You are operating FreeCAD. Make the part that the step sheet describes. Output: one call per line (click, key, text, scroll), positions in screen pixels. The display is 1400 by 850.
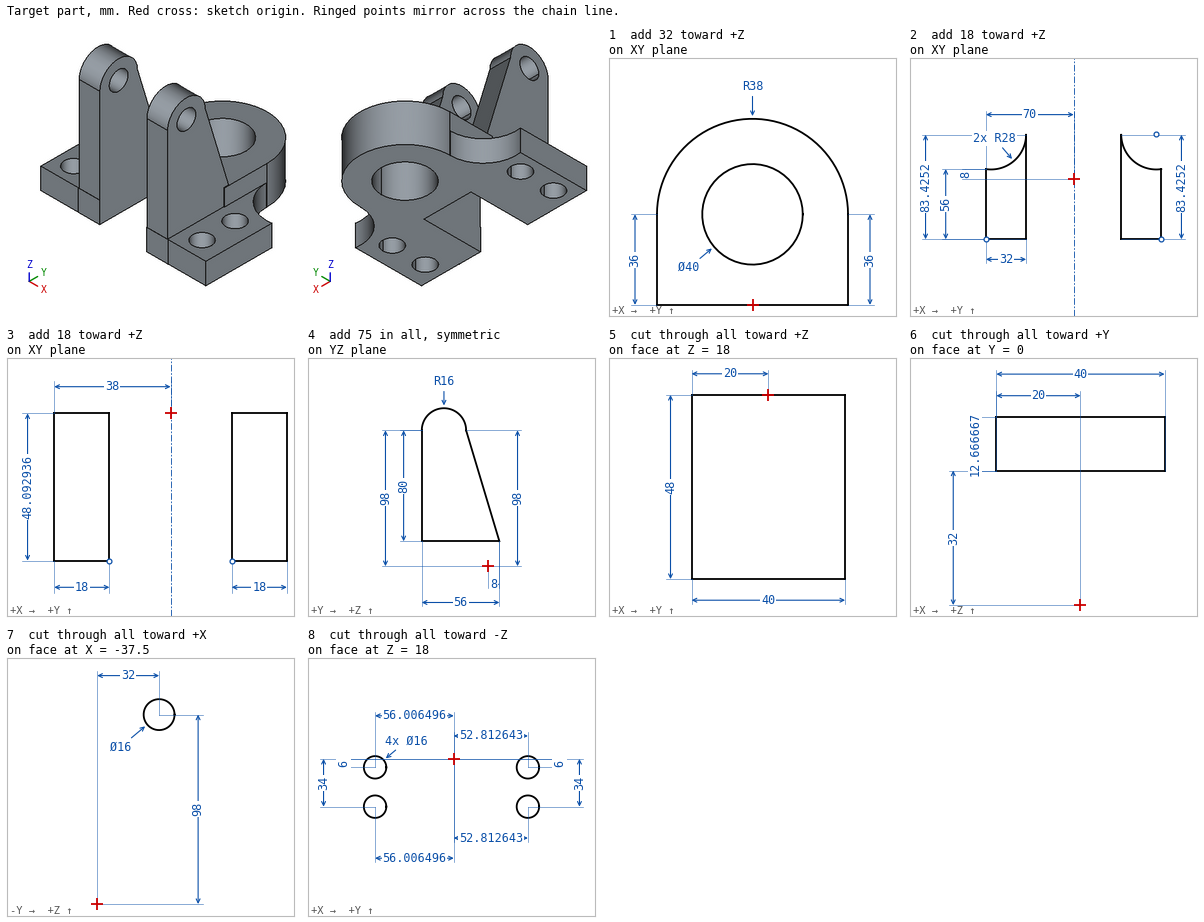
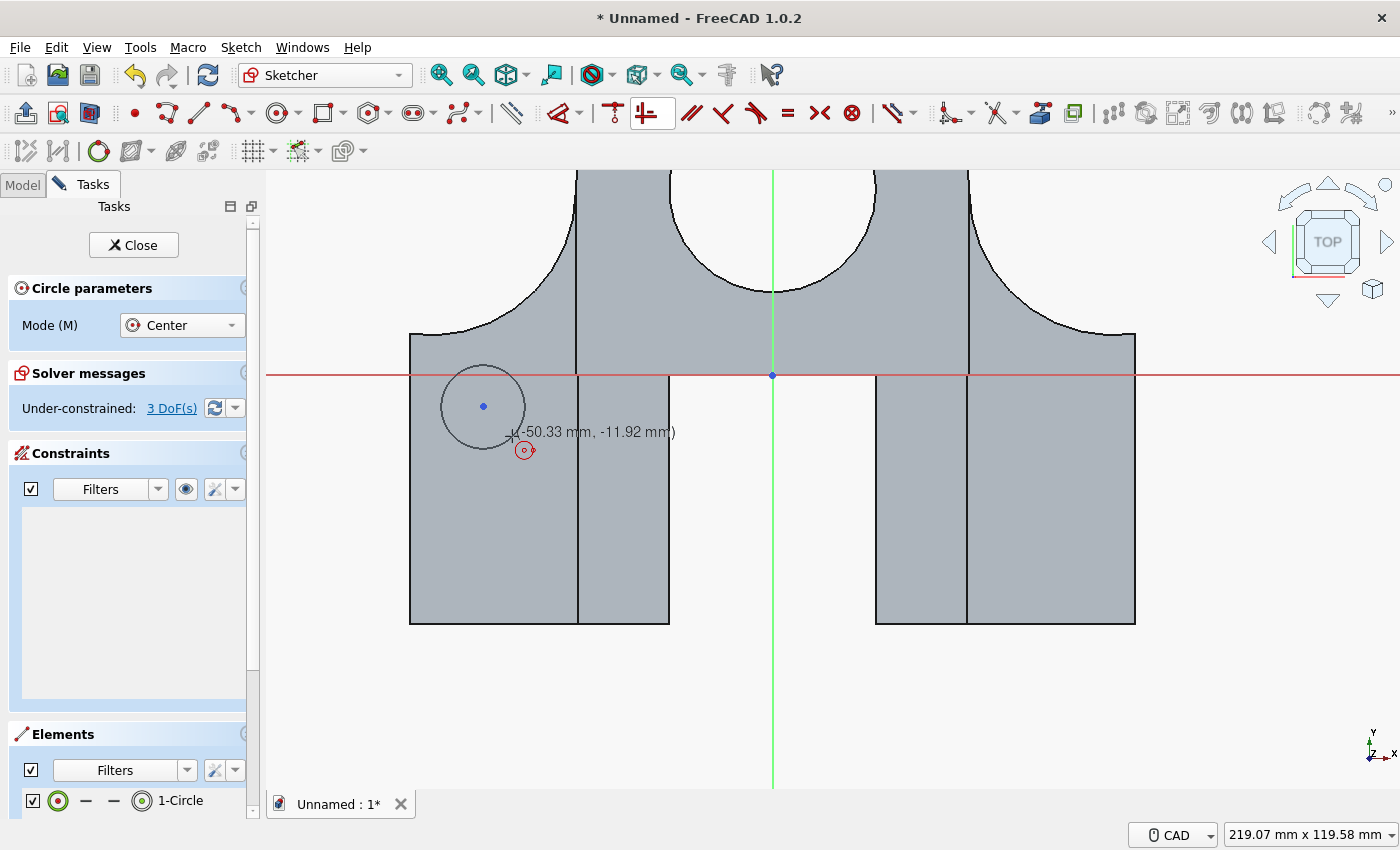
click(483, 551)
click(512, 522)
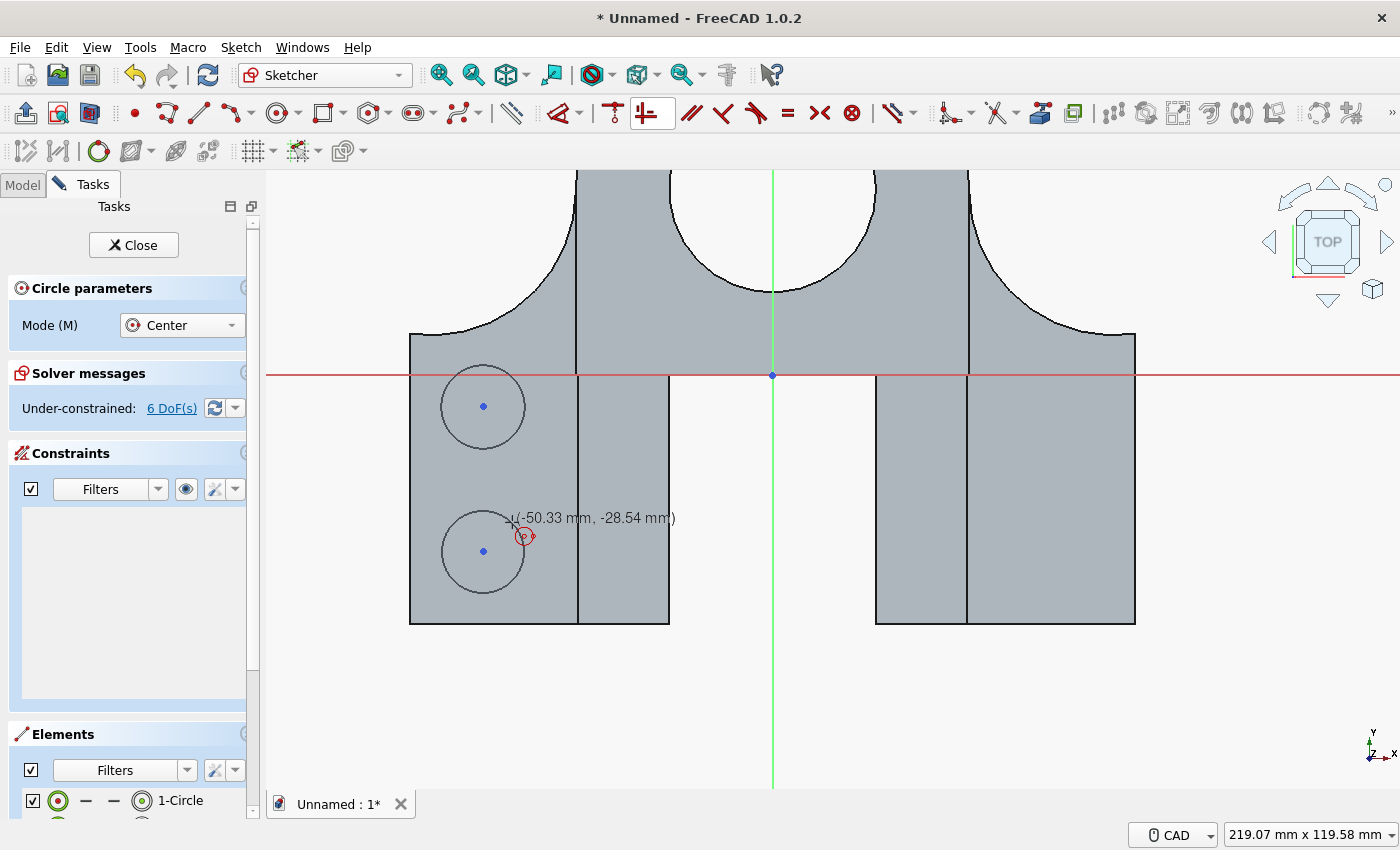
click(1046, 406)
click(1075, 436)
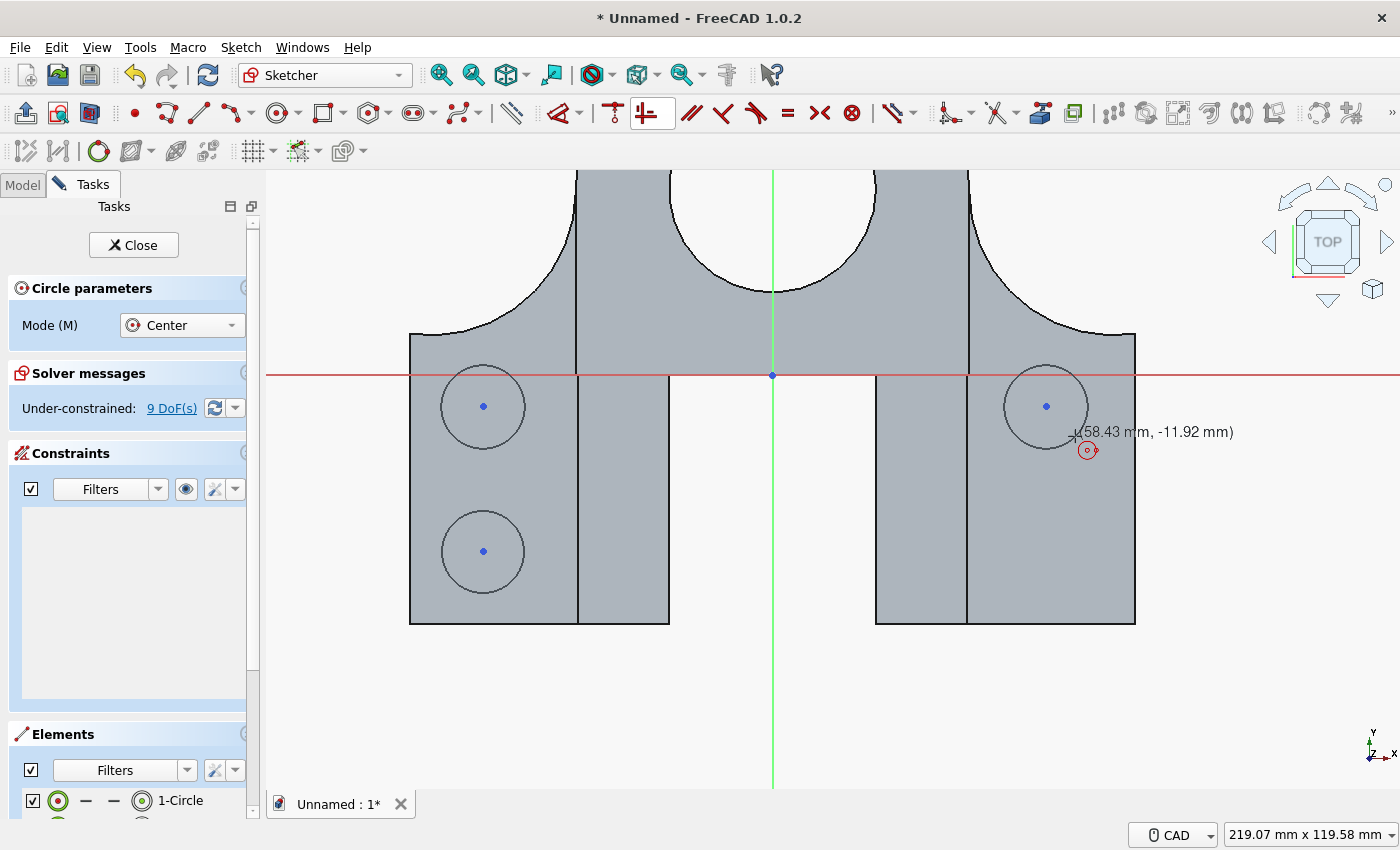
click(1046, 551)
click(1075, 522)
key(Escape)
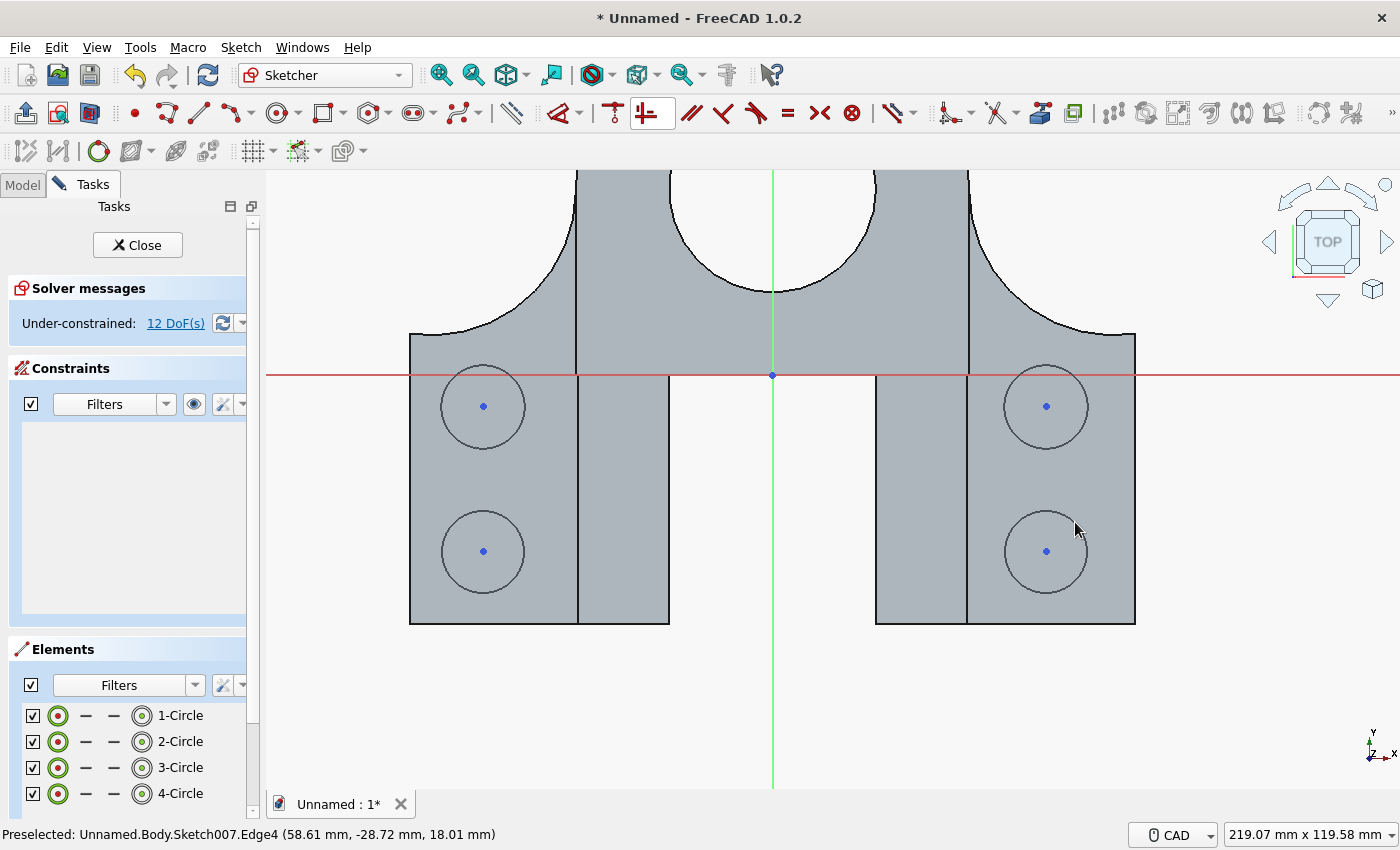
click(512, 377)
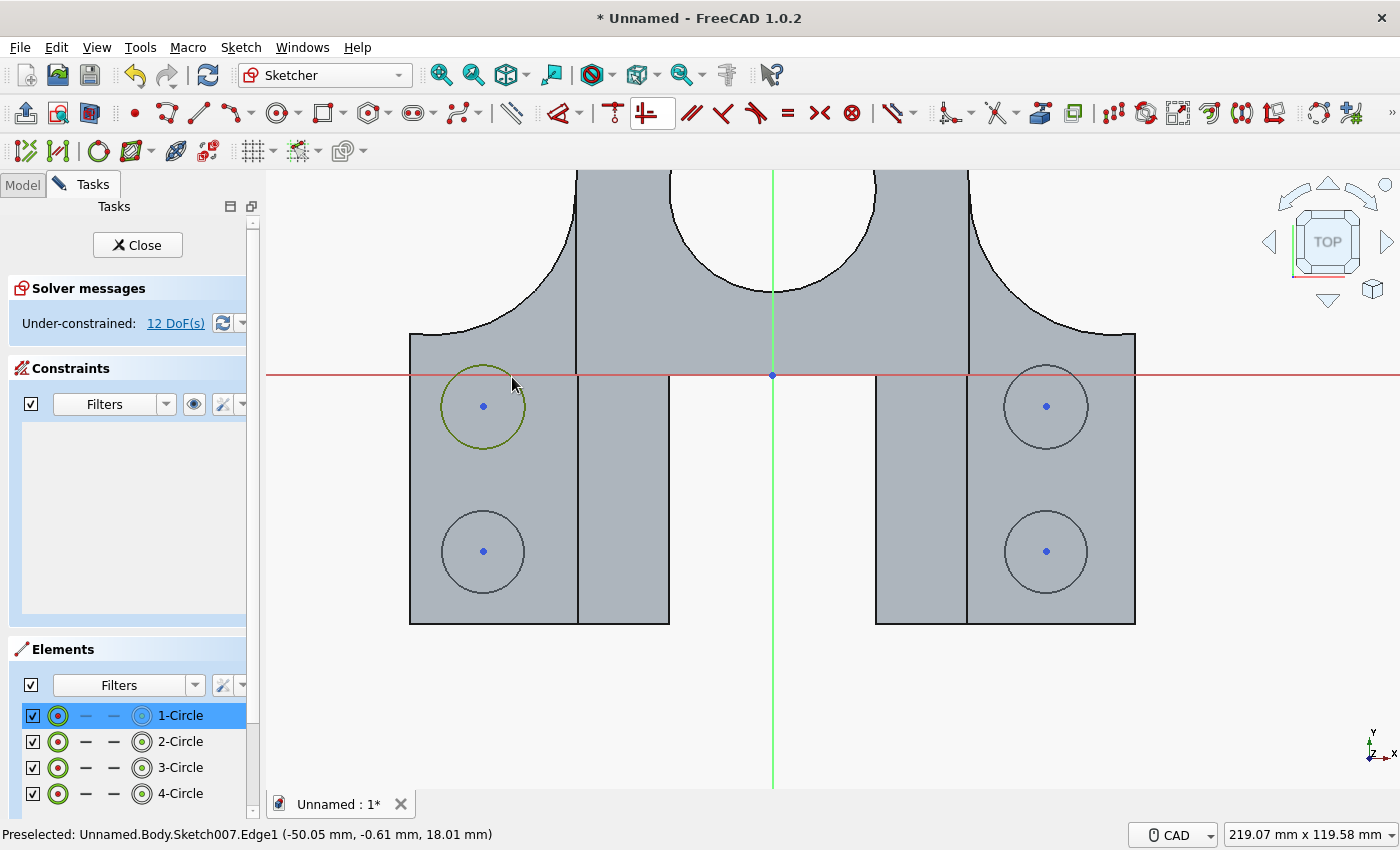
click(512, 523)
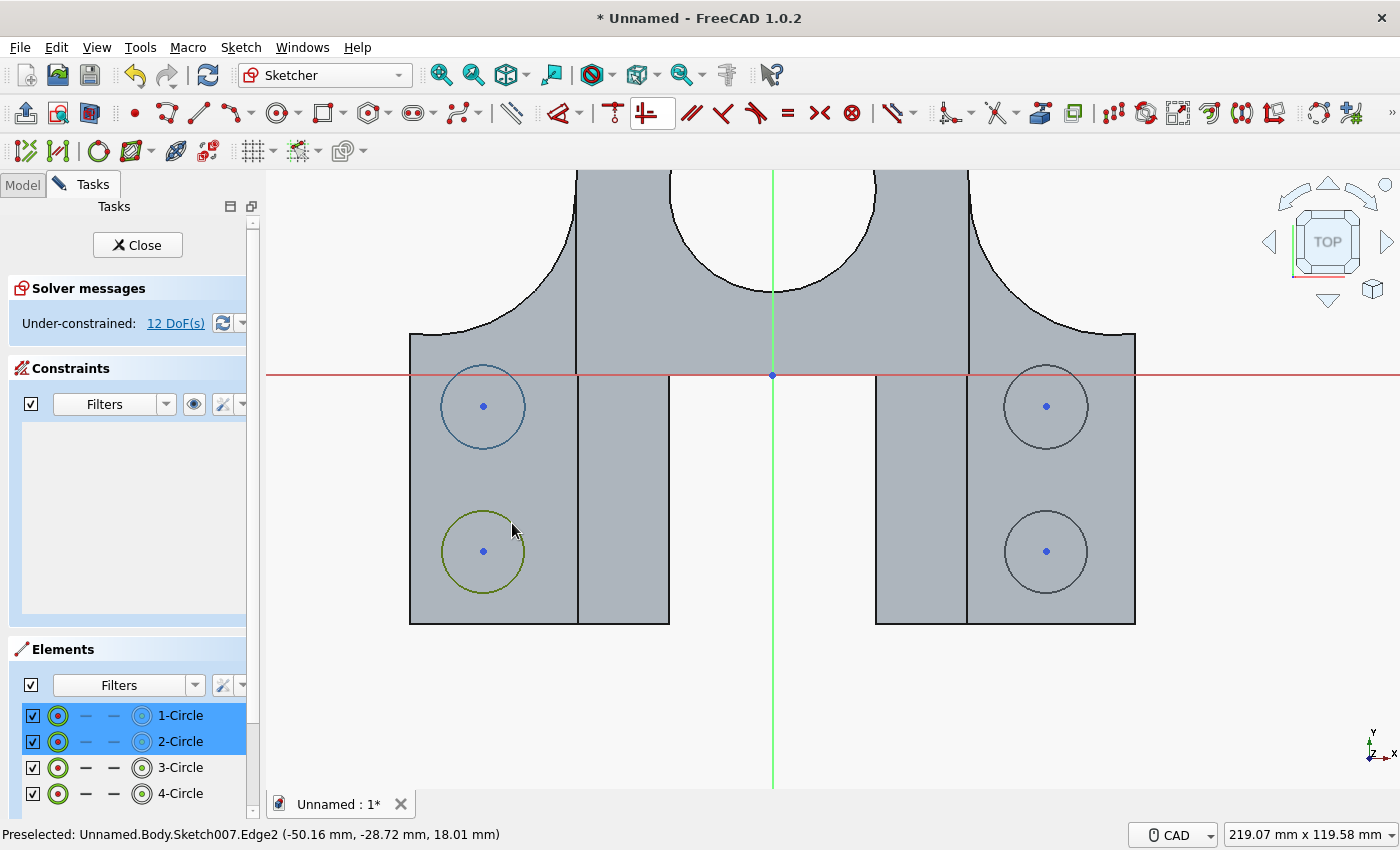
click(1075, 377)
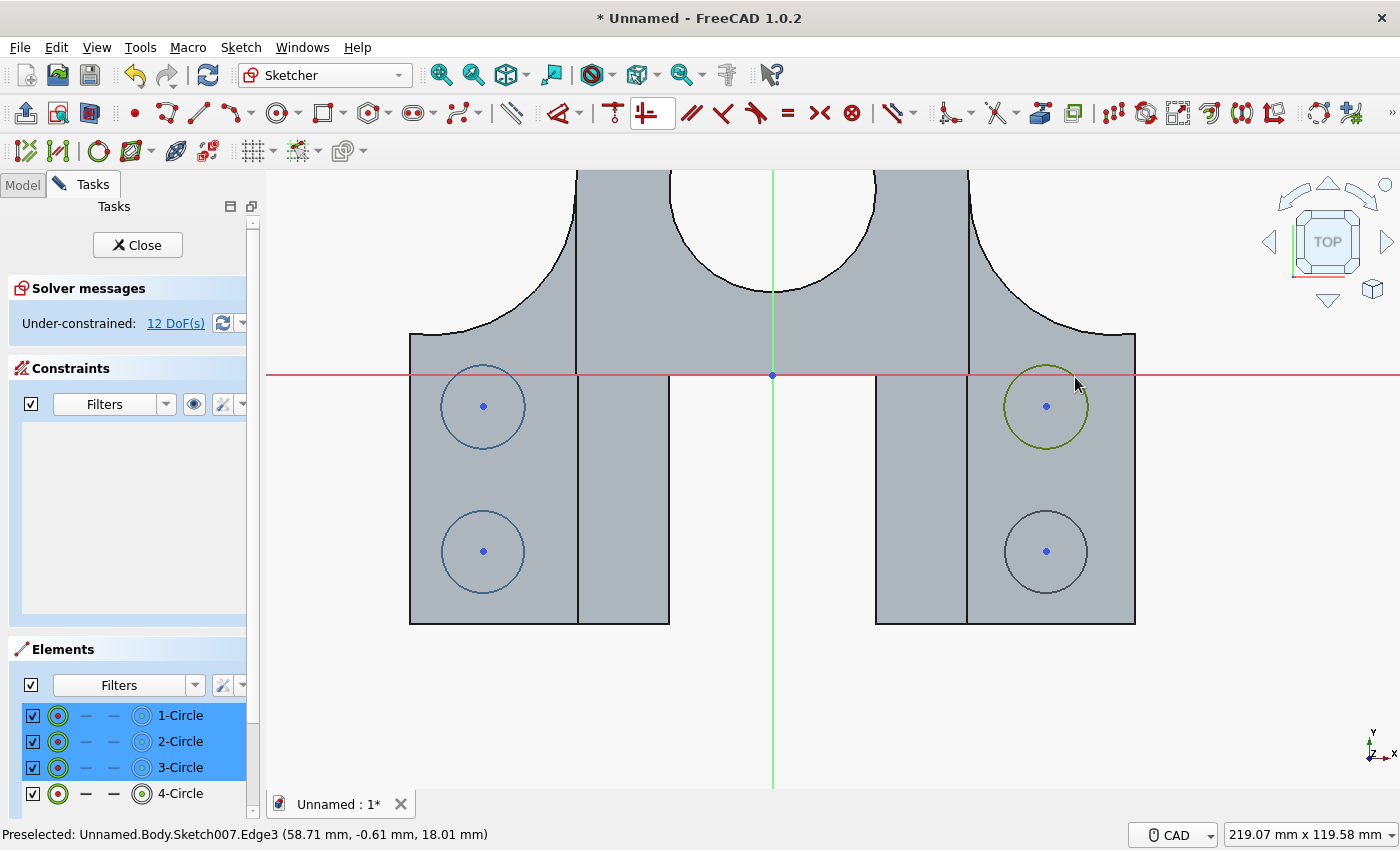
click(1075, 523)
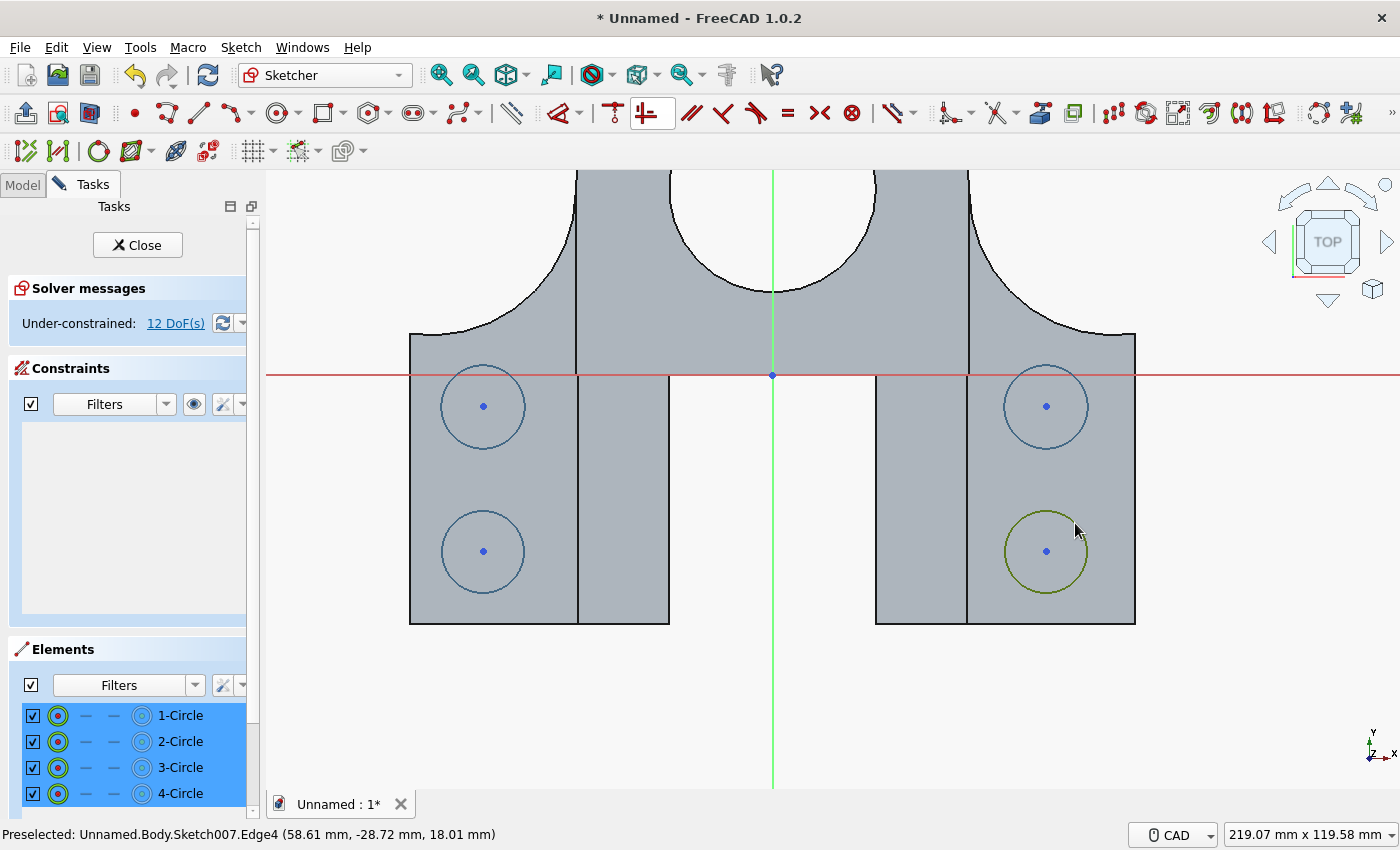
click(788, 114)